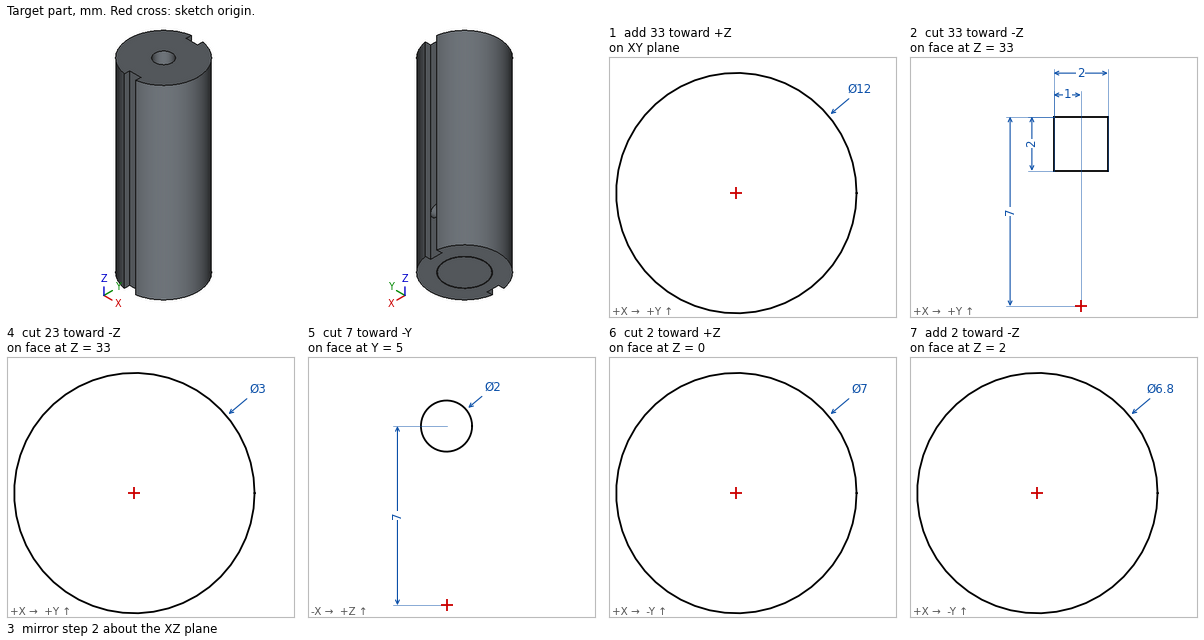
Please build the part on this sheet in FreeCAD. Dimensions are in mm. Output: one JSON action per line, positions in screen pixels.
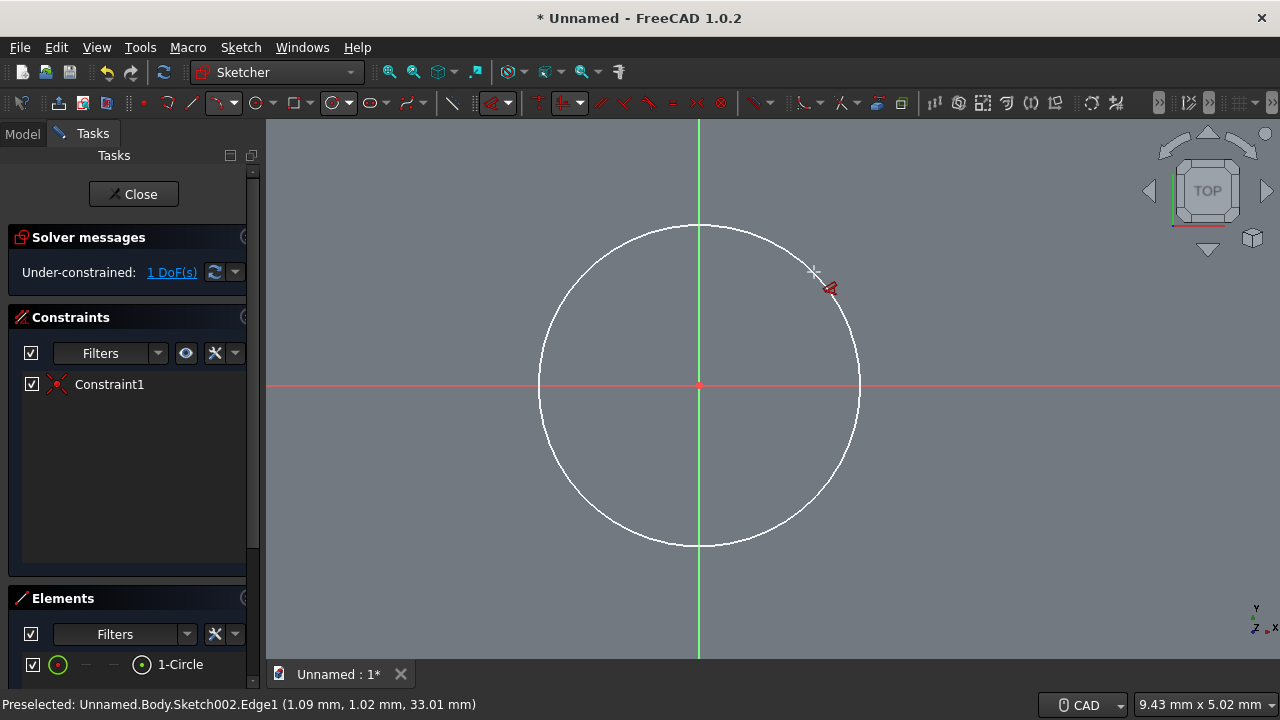
{"action": "left_click", "coordinate": [813, 272]}
{"action": "left_click", "coordinate": [836, 249]}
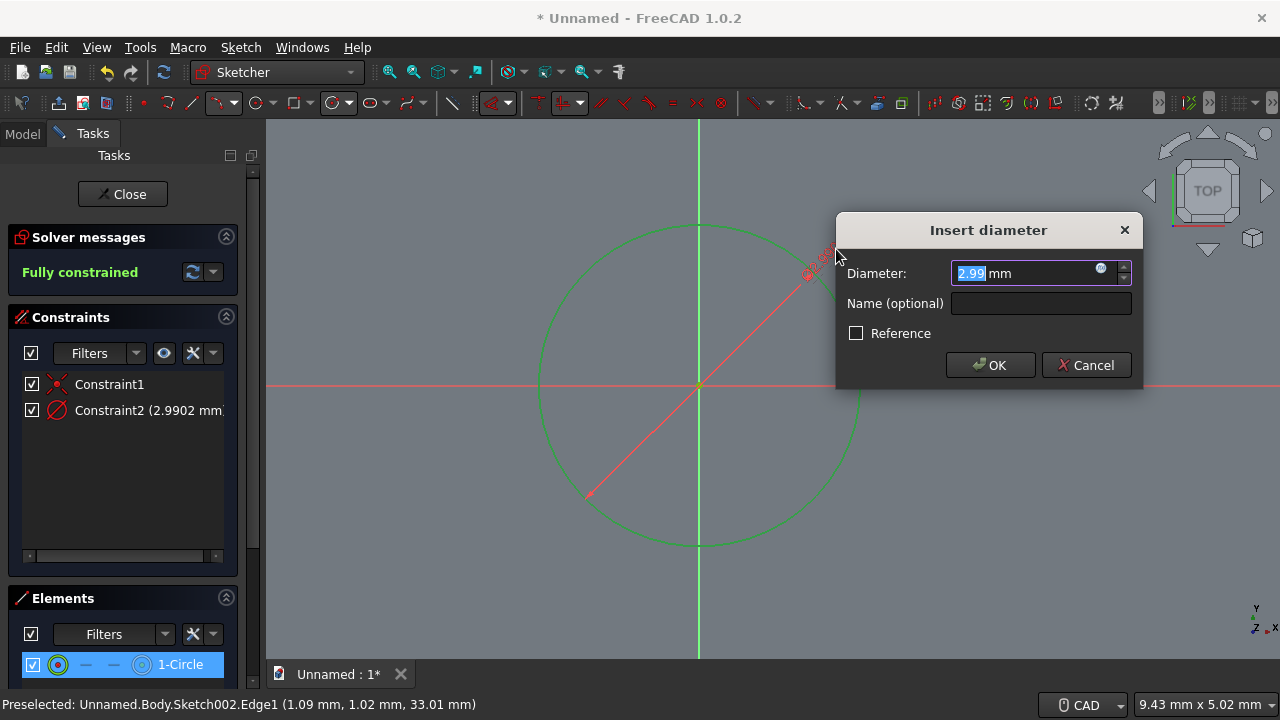
{"action": "type", "text": "3"}
{"action": "key", "text": "Return"}
{"action": "key", "text": "Escape"}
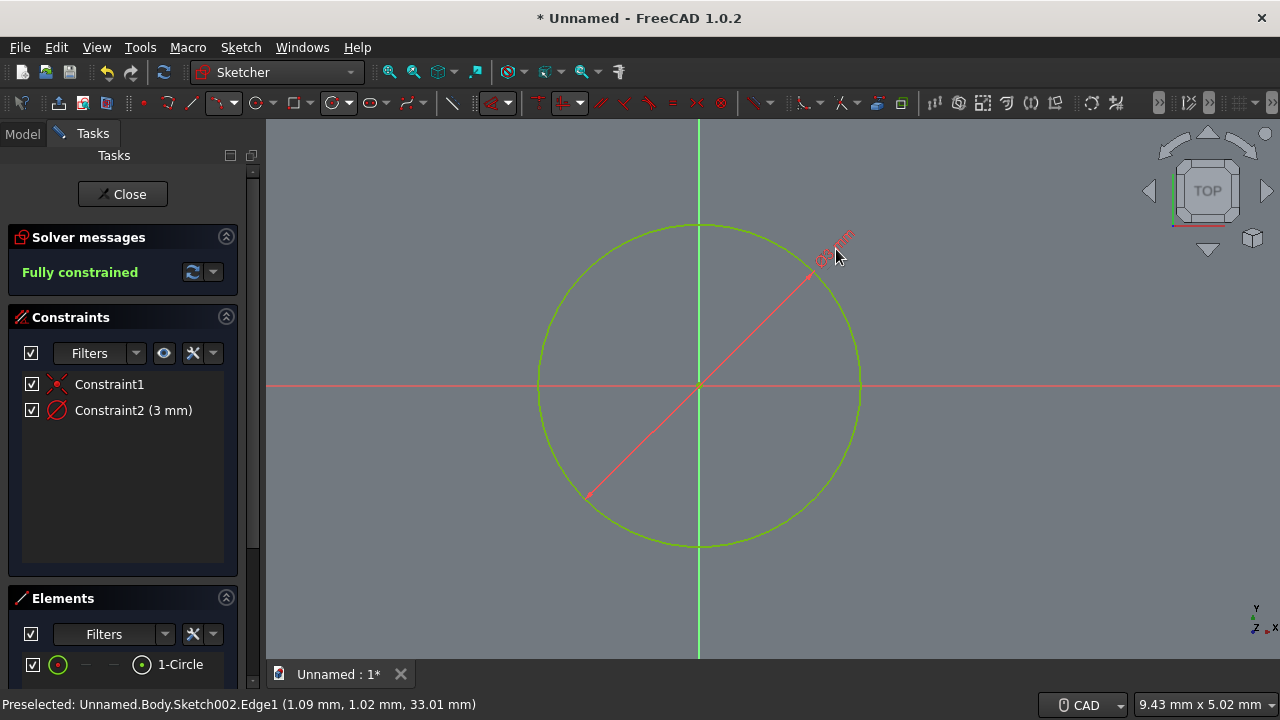
{"action": "left_click", "coordinate": [123, 194]}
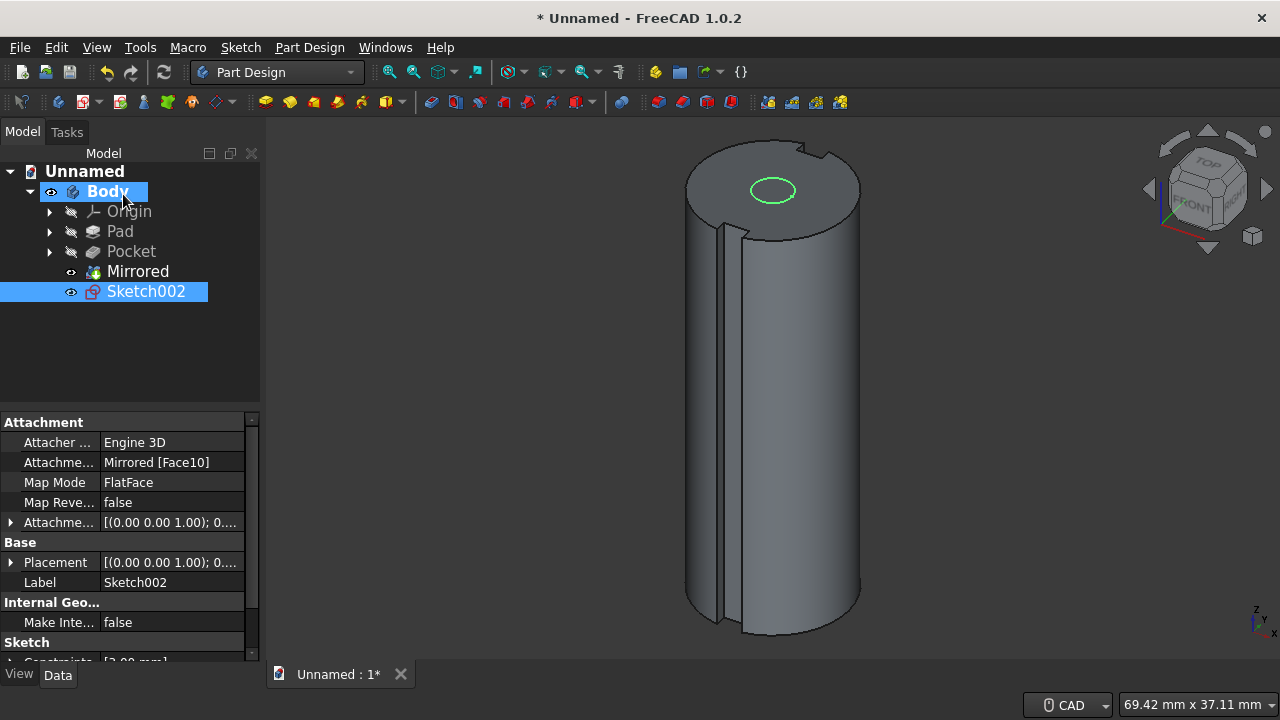
{"action": "left_click", "coordinate": [432, 102]}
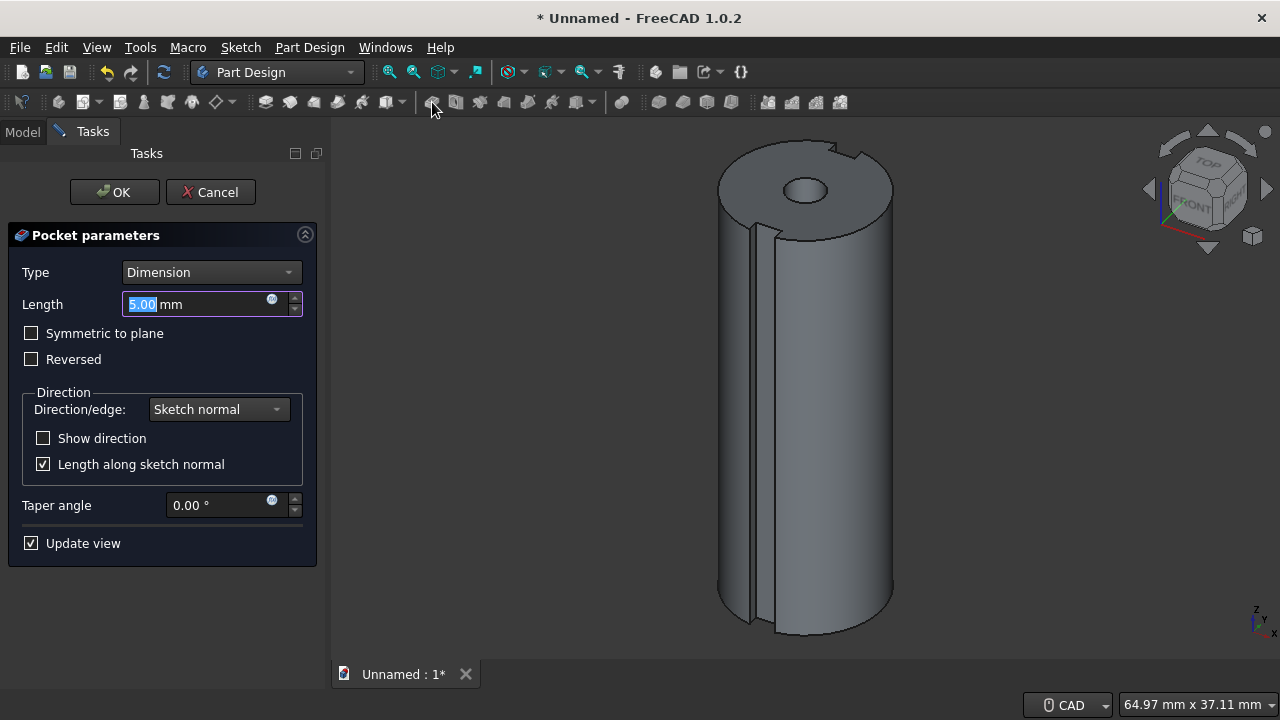
{"action": "type", "text": "23"}
{"action": "key", "text": "Tab"}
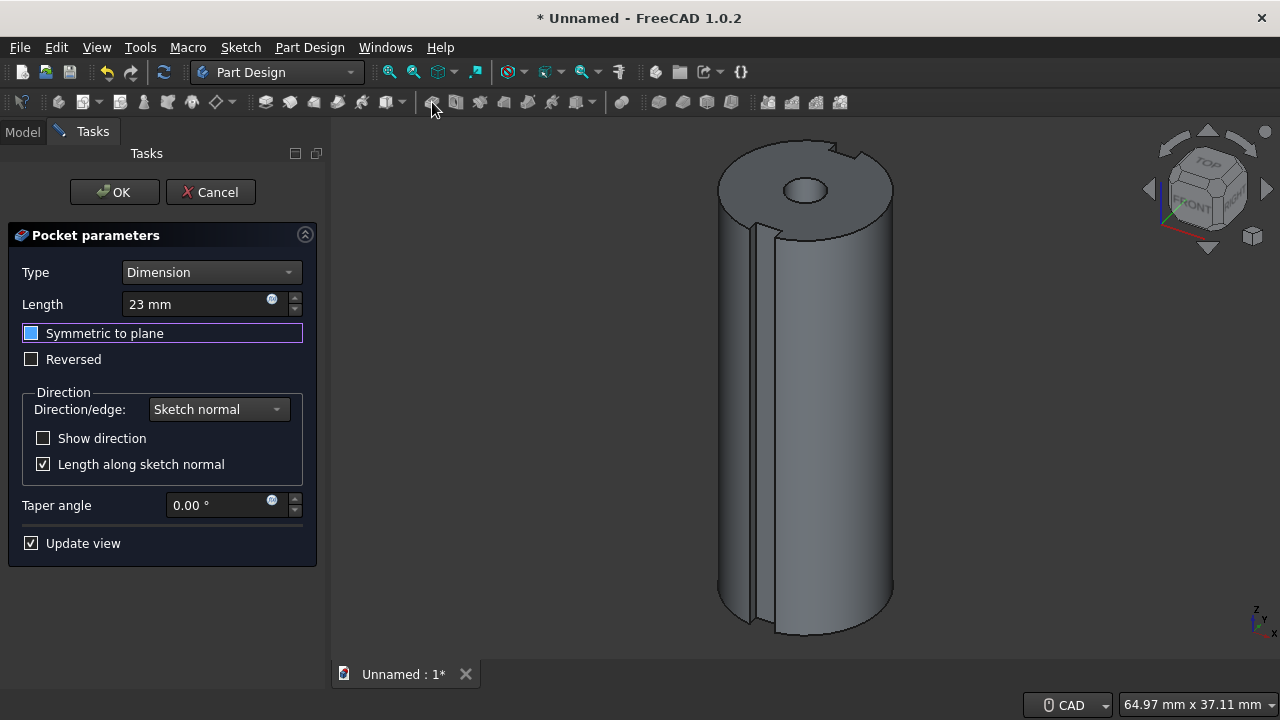
{"action": "left_click", "coordinate": [115, 192]}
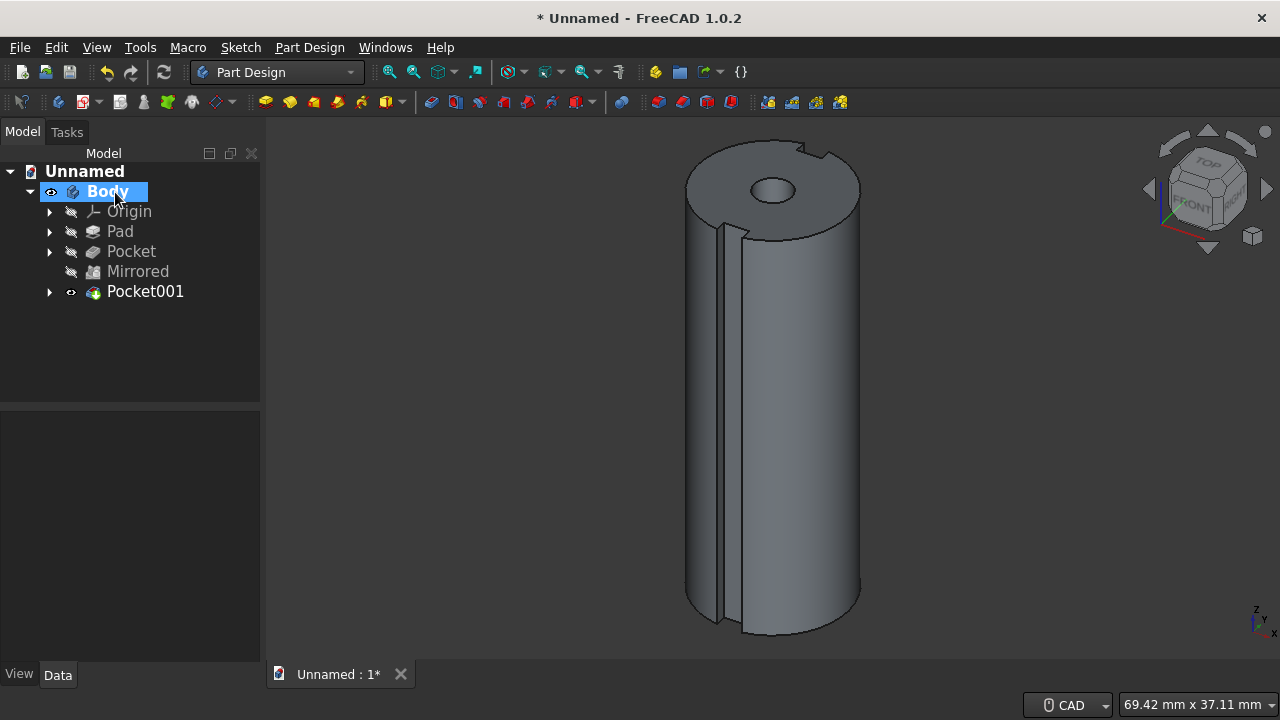
{"action": "key", "text": "4"}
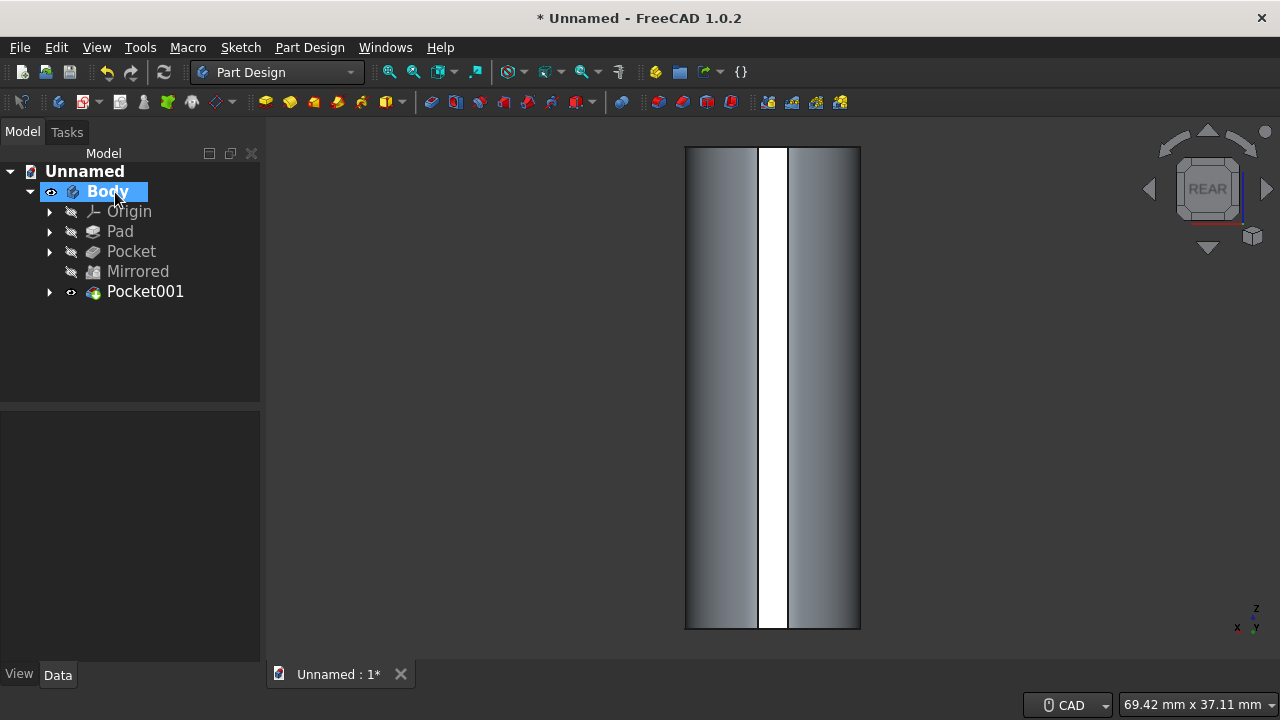
{"action": "left_click", "coordinate": [773, 180]}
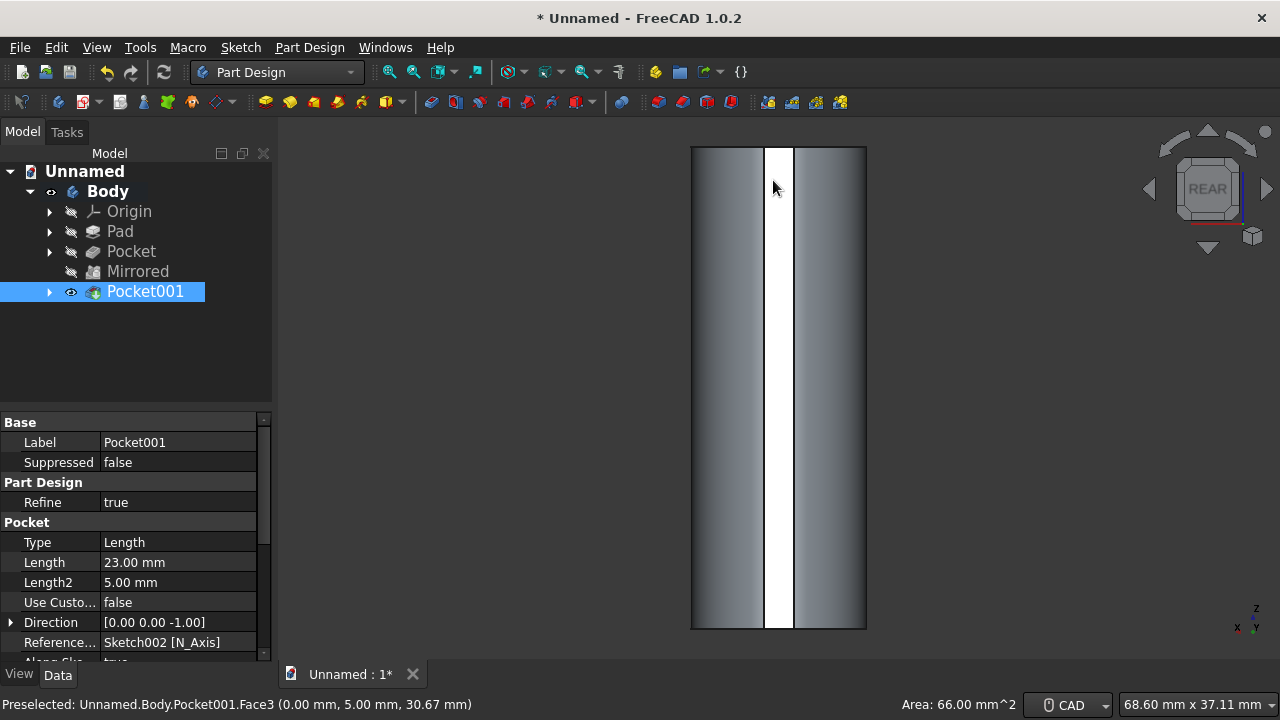
{"action": "left_click", "coordinate": [84, 102]}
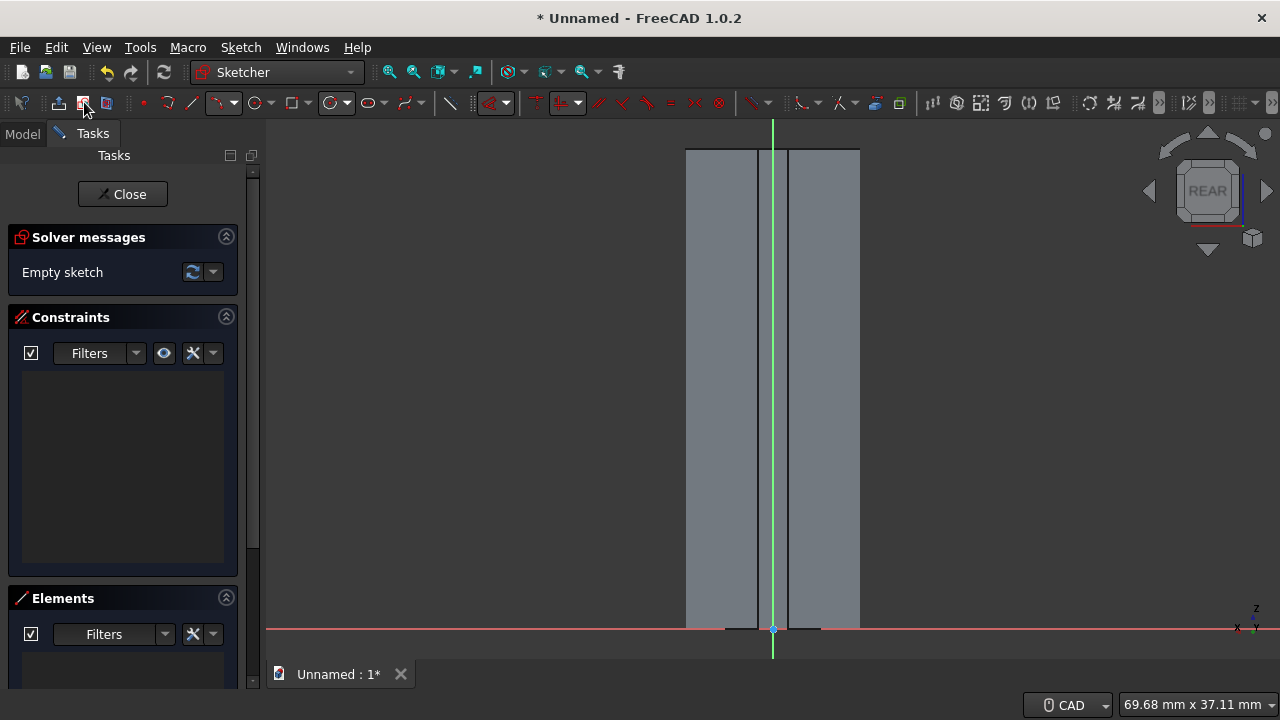
{"action": "left_click", "coordinate": [108, 104]}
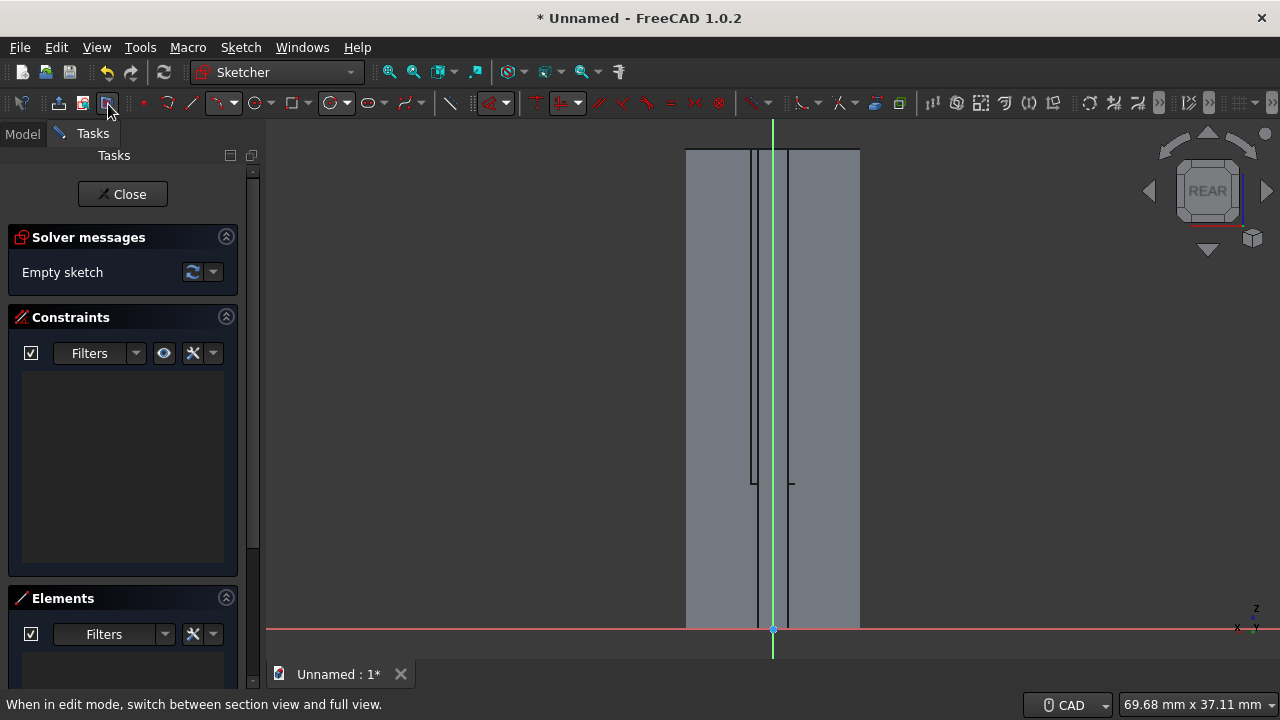
{"action": "scroll", "coordinate": [780, 541], "scroll_direction": "up", "scroll_amount": 12}